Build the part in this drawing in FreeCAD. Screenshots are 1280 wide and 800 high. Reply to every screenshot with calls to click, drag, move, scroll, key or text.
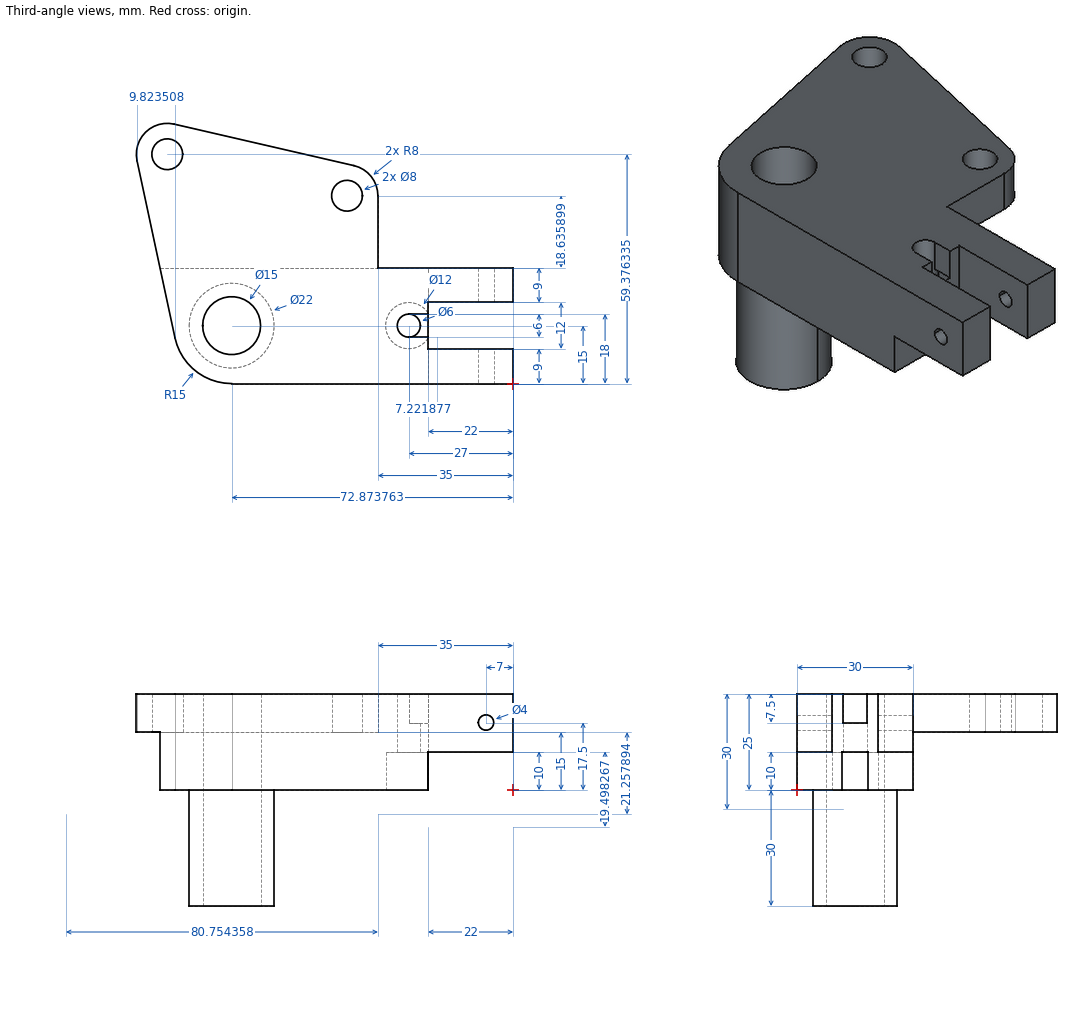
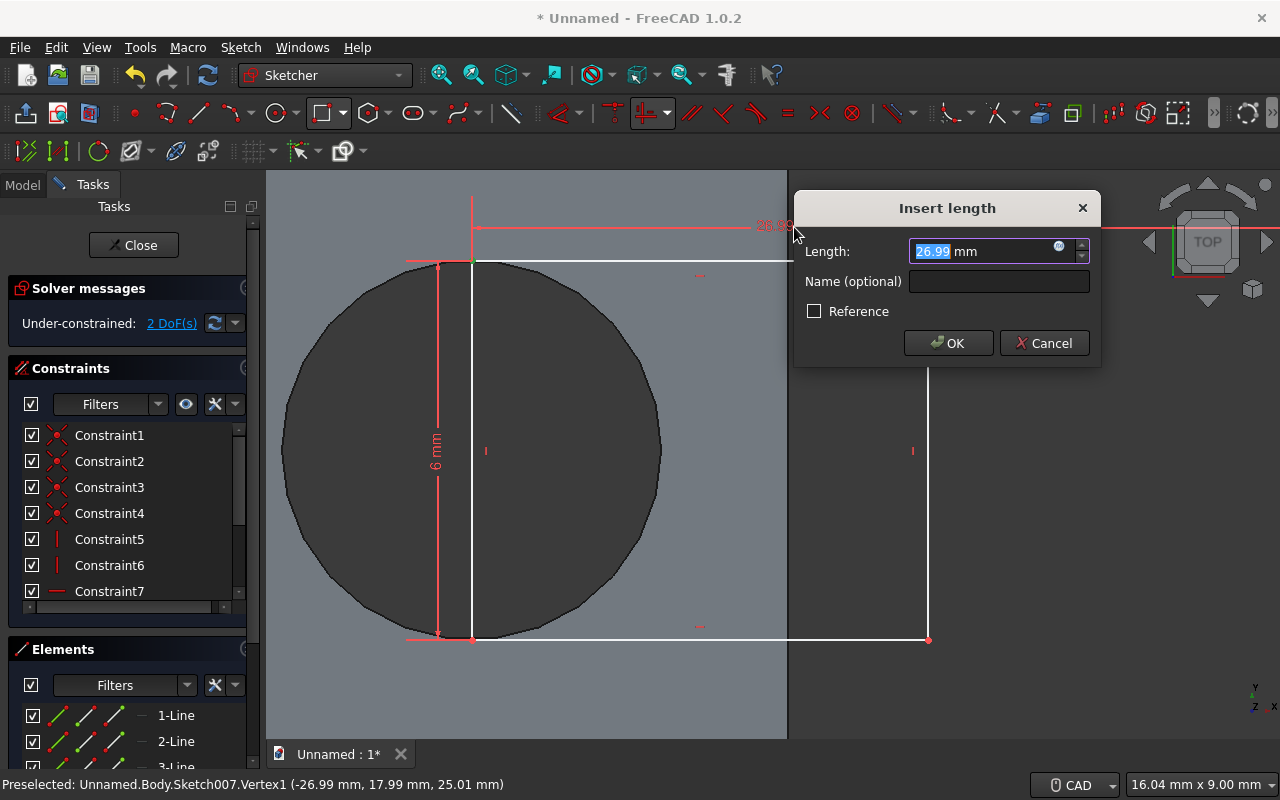
text(27)
key(Return)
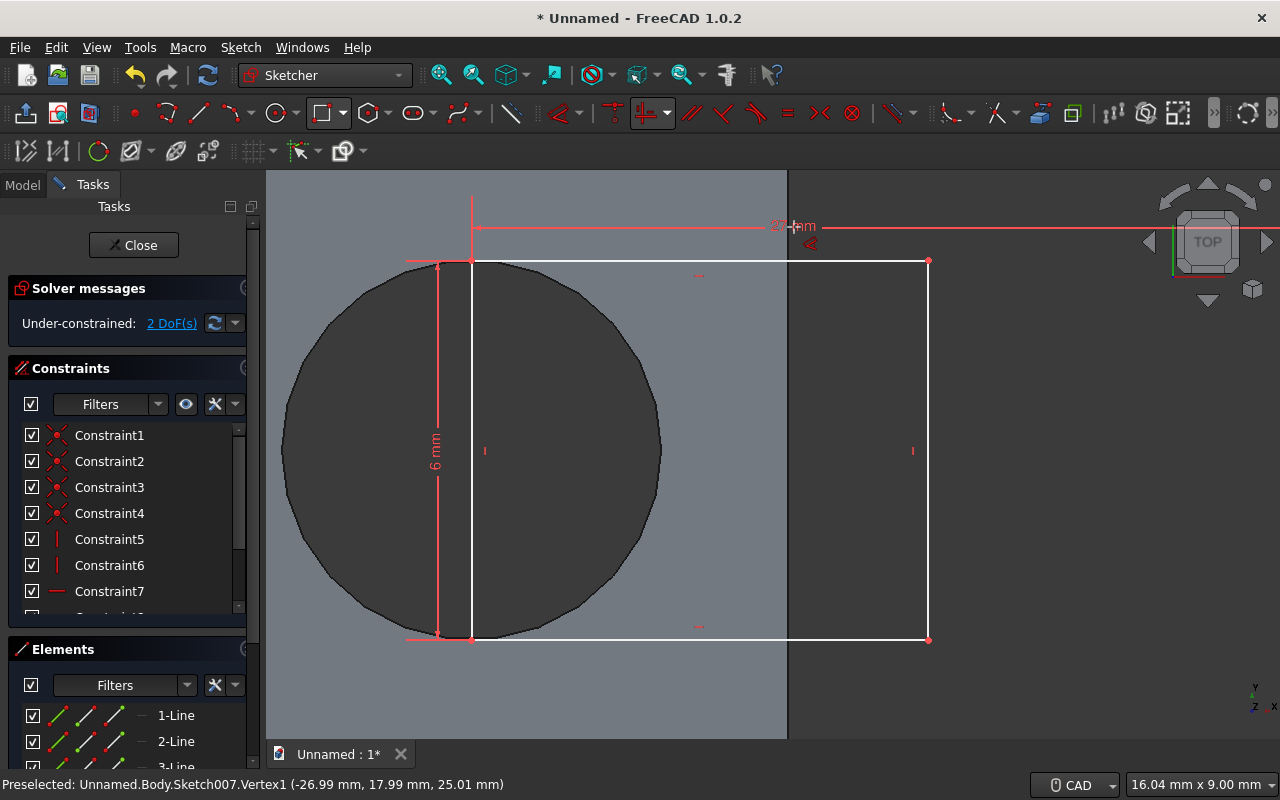
click(472, 261)
click(438, 486)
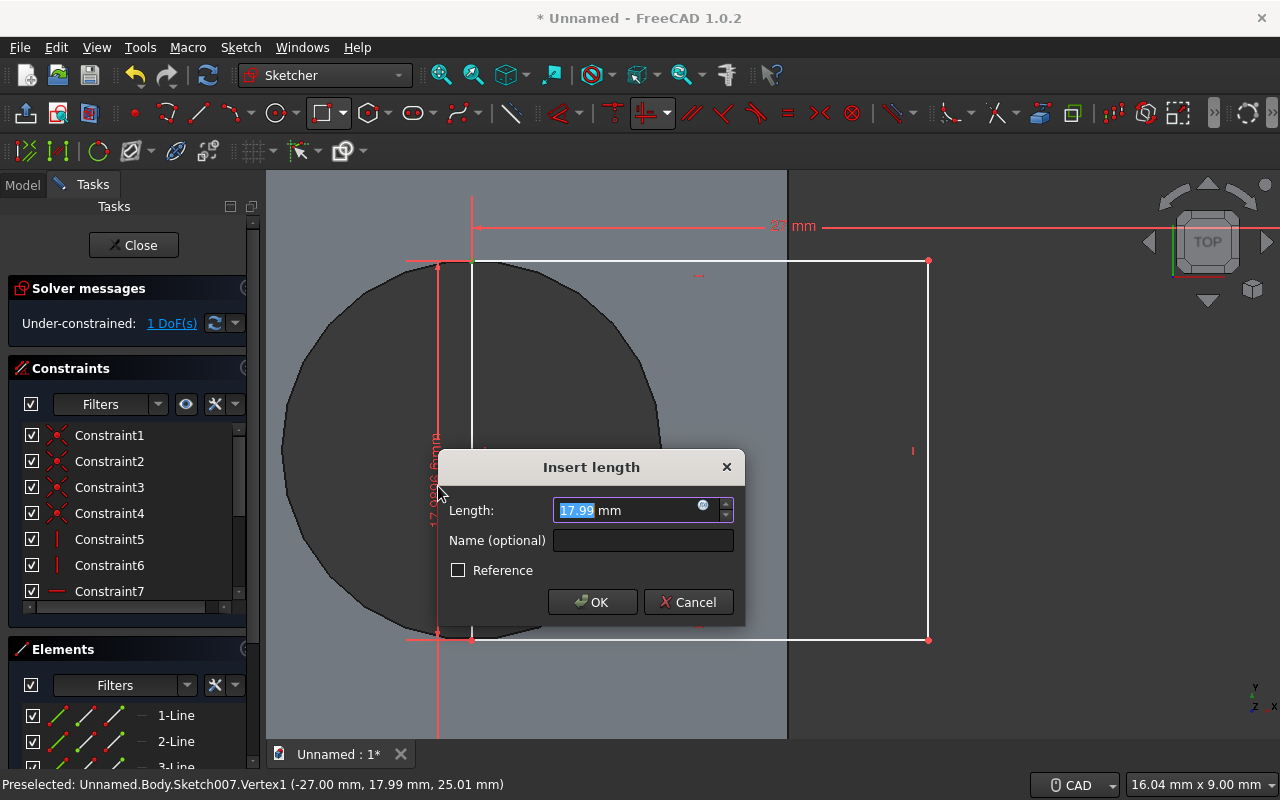
text(18)
key(Return)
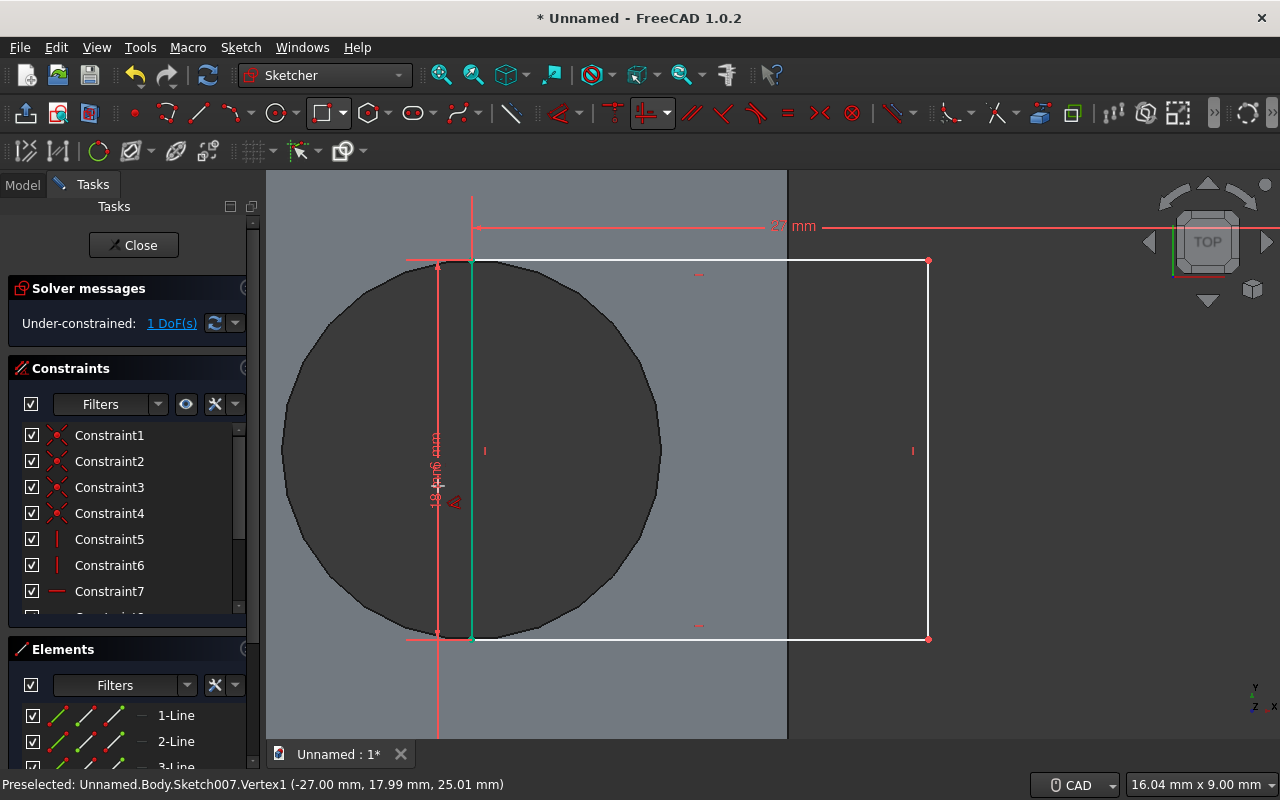
click(608, 640)
click(700, 674)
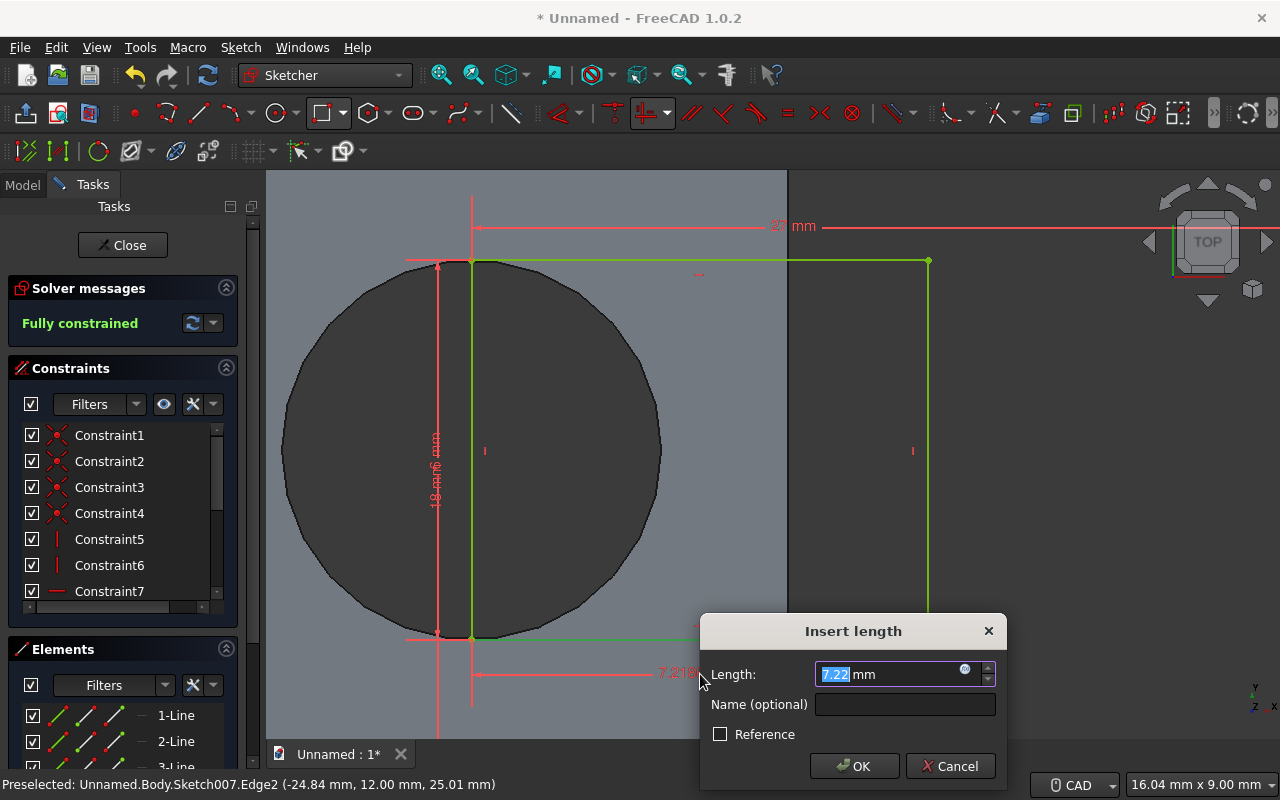
text(7.221877)
key(Return)
key(Escape)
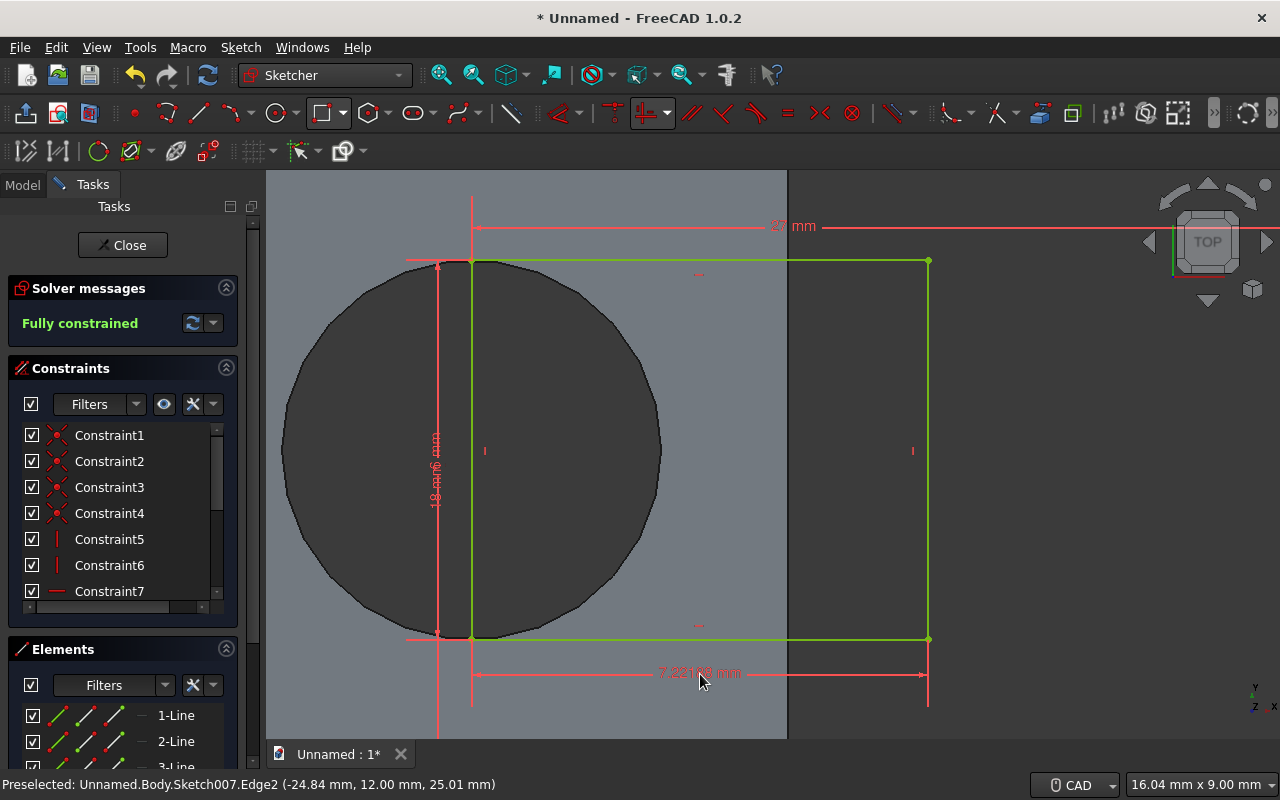
click(123, 245)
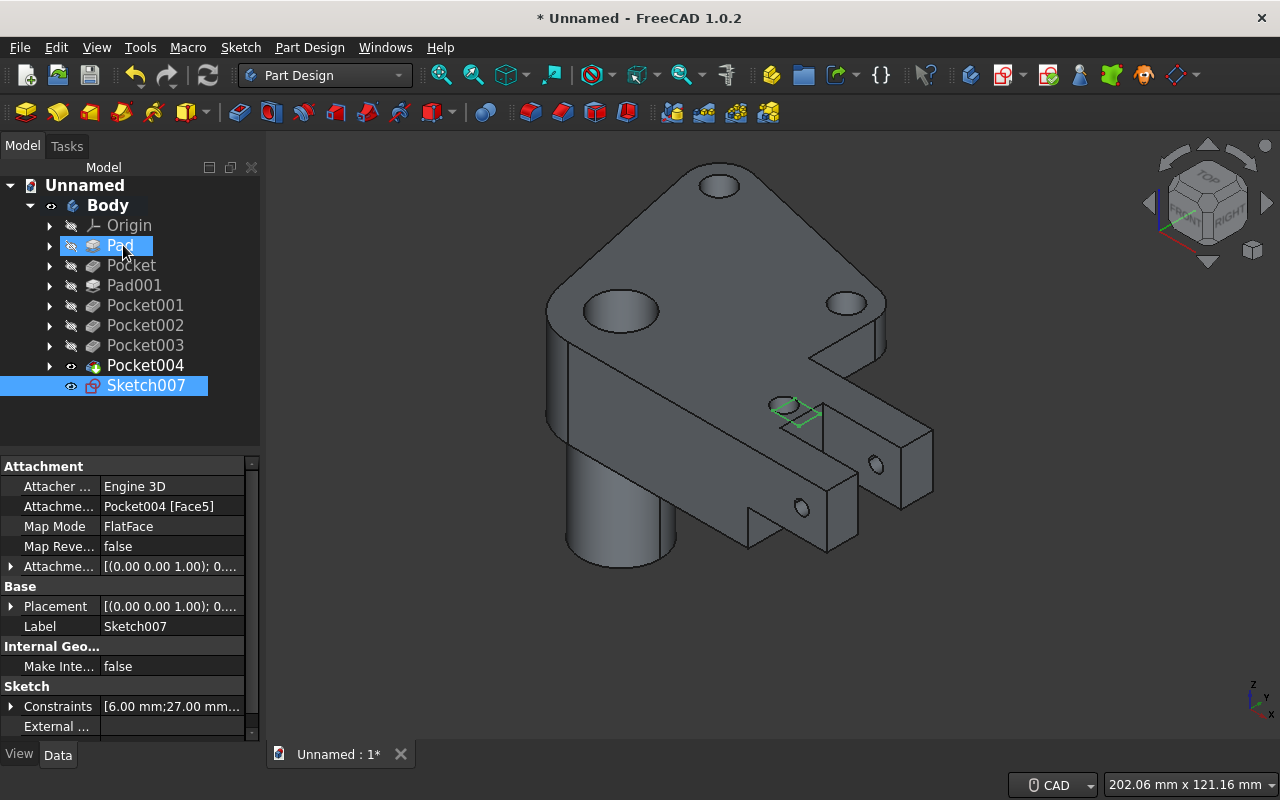
click(240, 112)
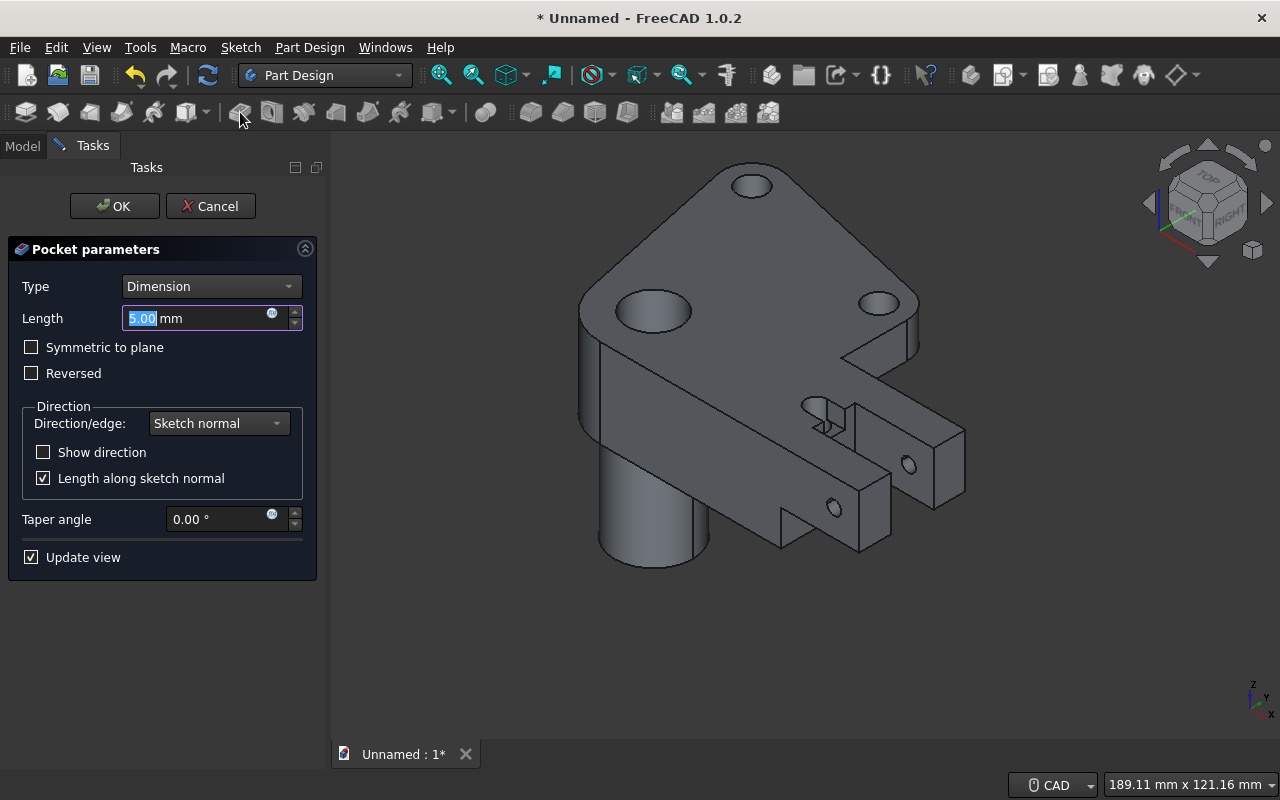
text(7.5)
key(Tab)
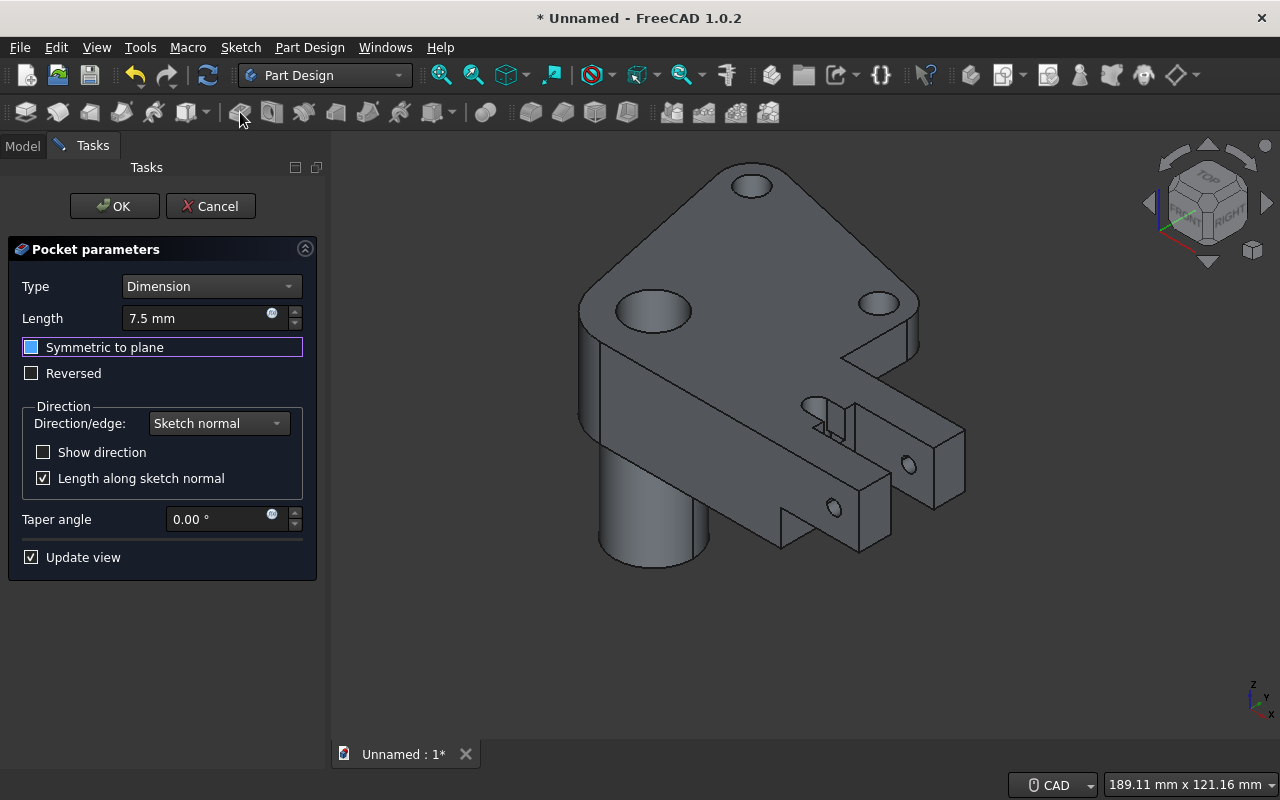
click(115, 206)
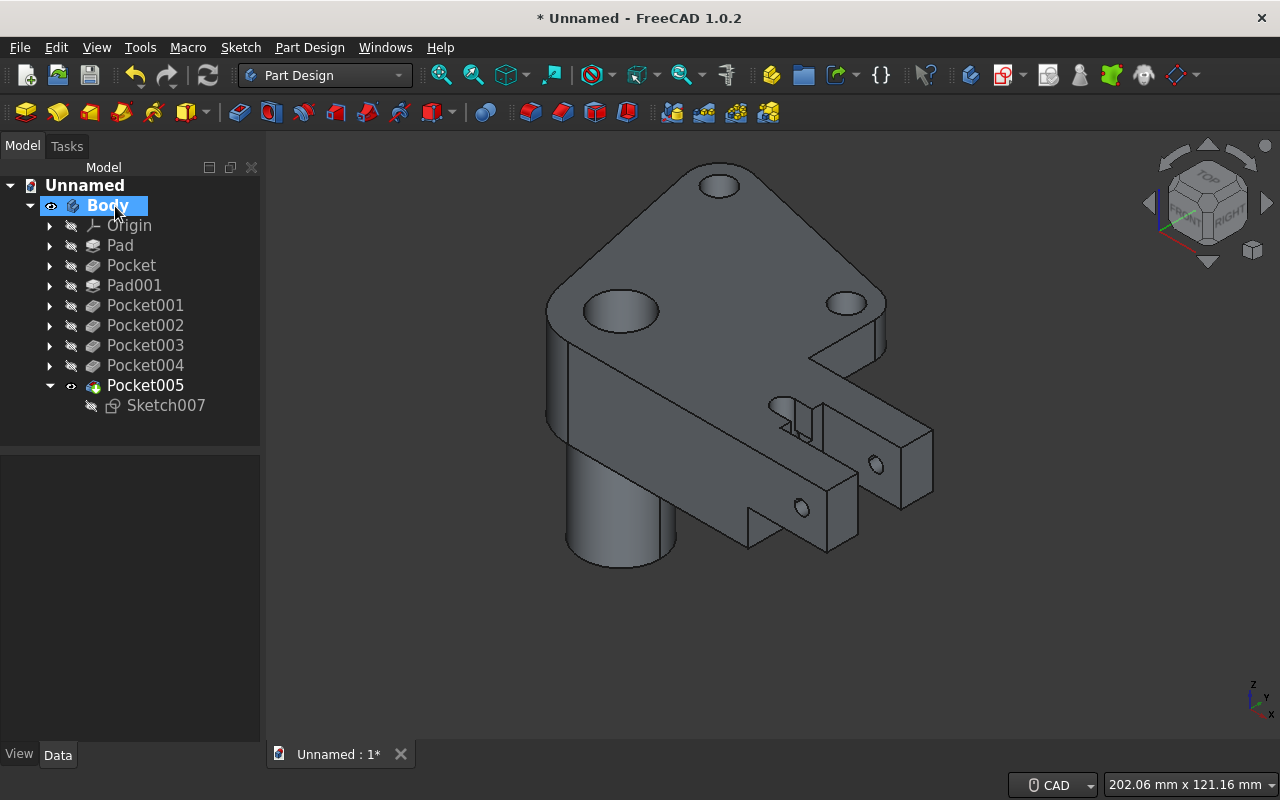
click(1004, 76)